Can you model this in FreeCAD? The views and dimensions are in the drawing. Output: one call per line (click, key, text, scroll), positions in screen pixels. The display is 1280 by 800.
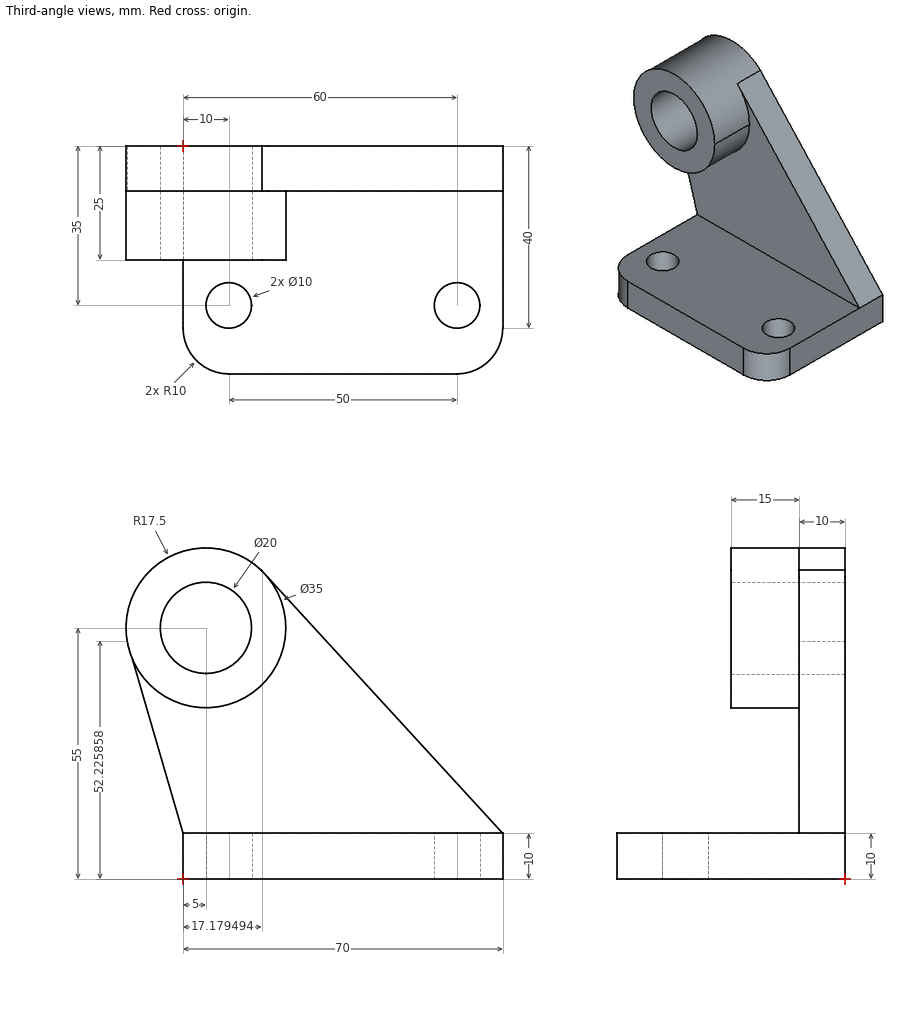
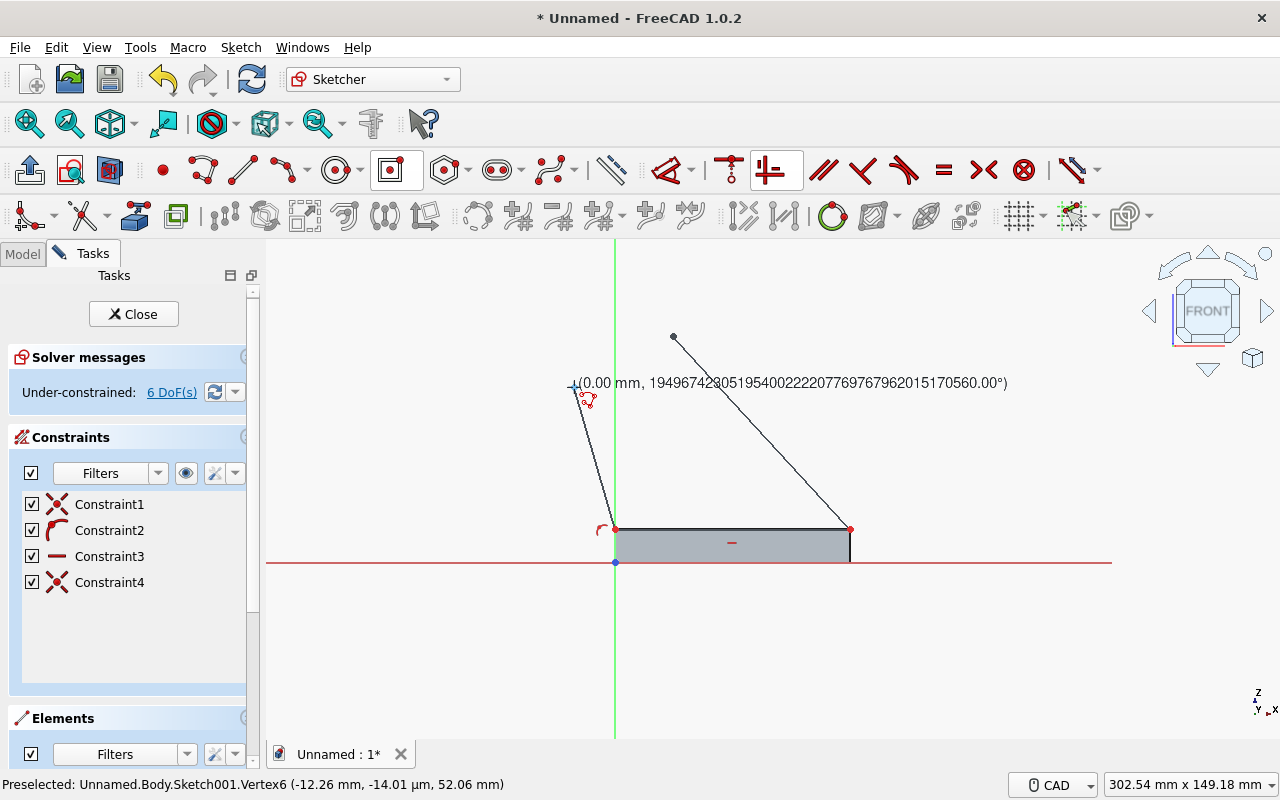
click(284, 170)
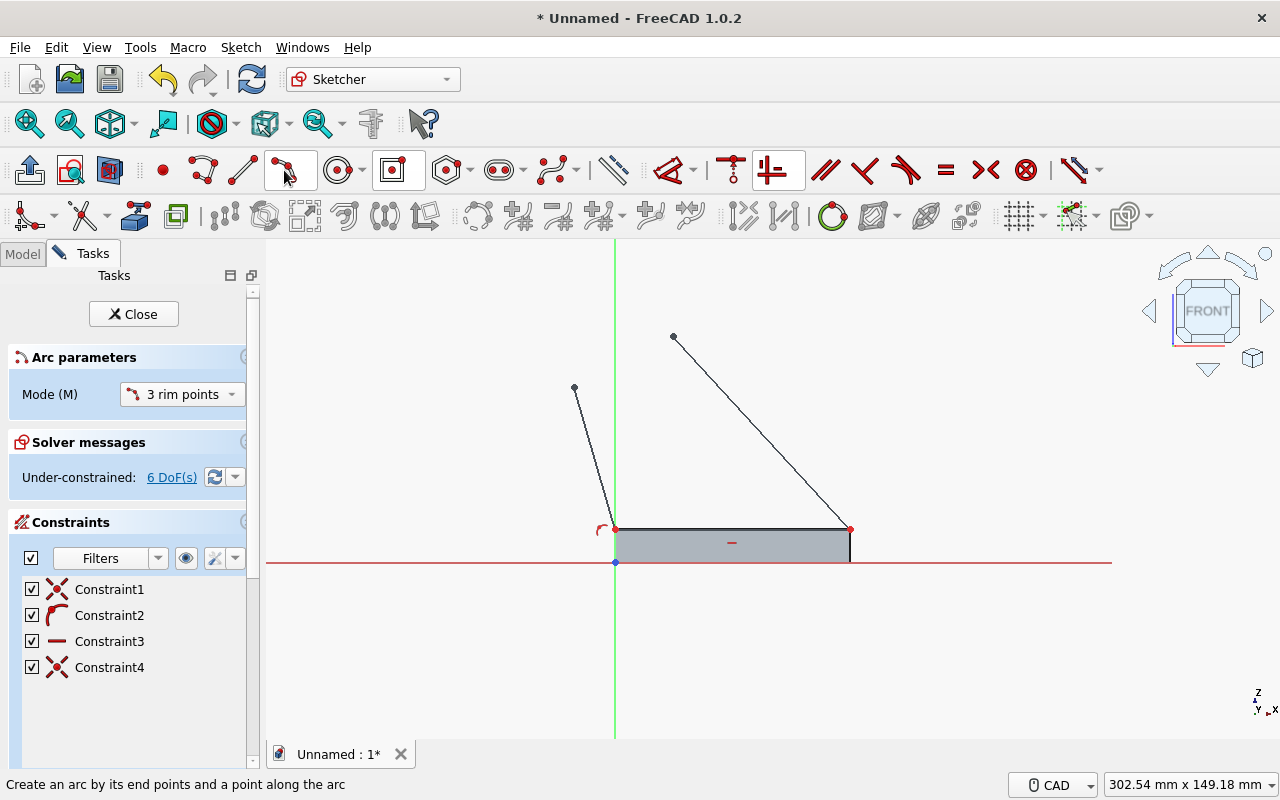
click(574, 388)
click(673, 337)
click(593, 334)
key(Escape)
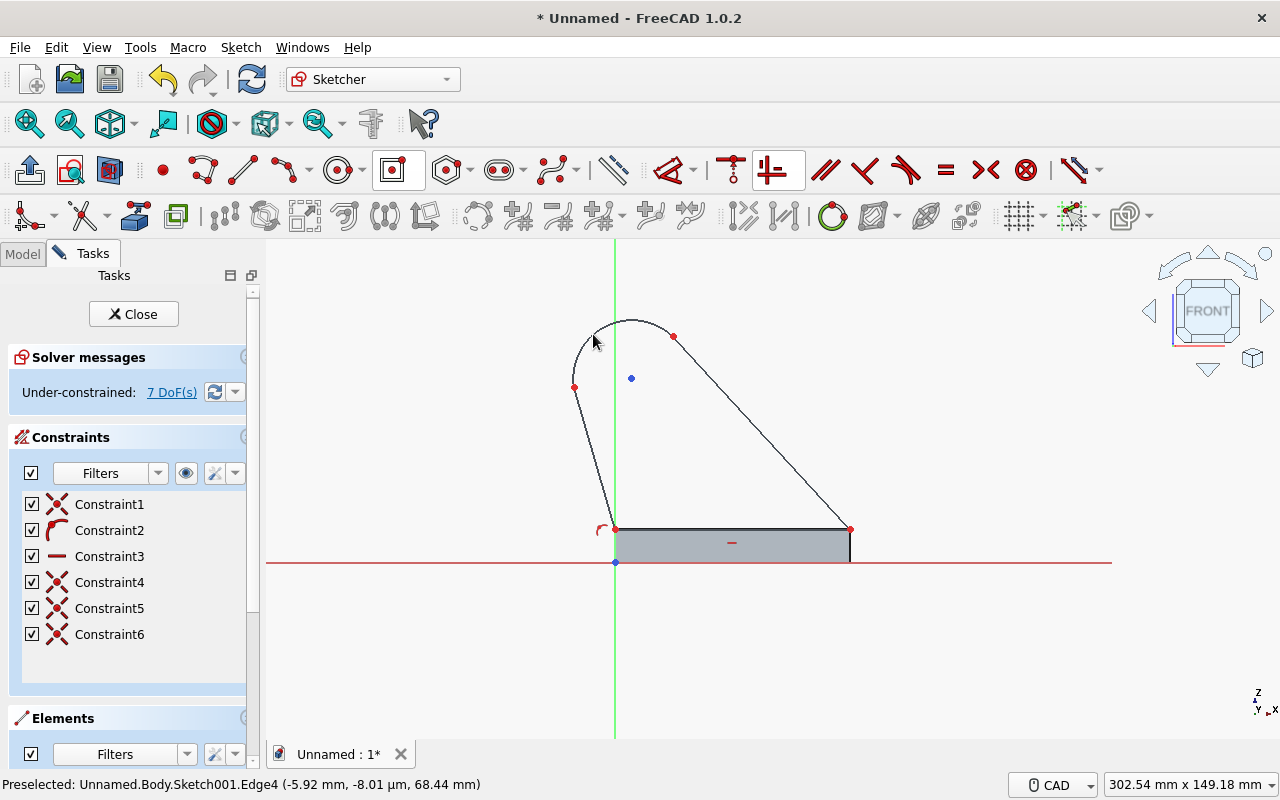
click(668, 170)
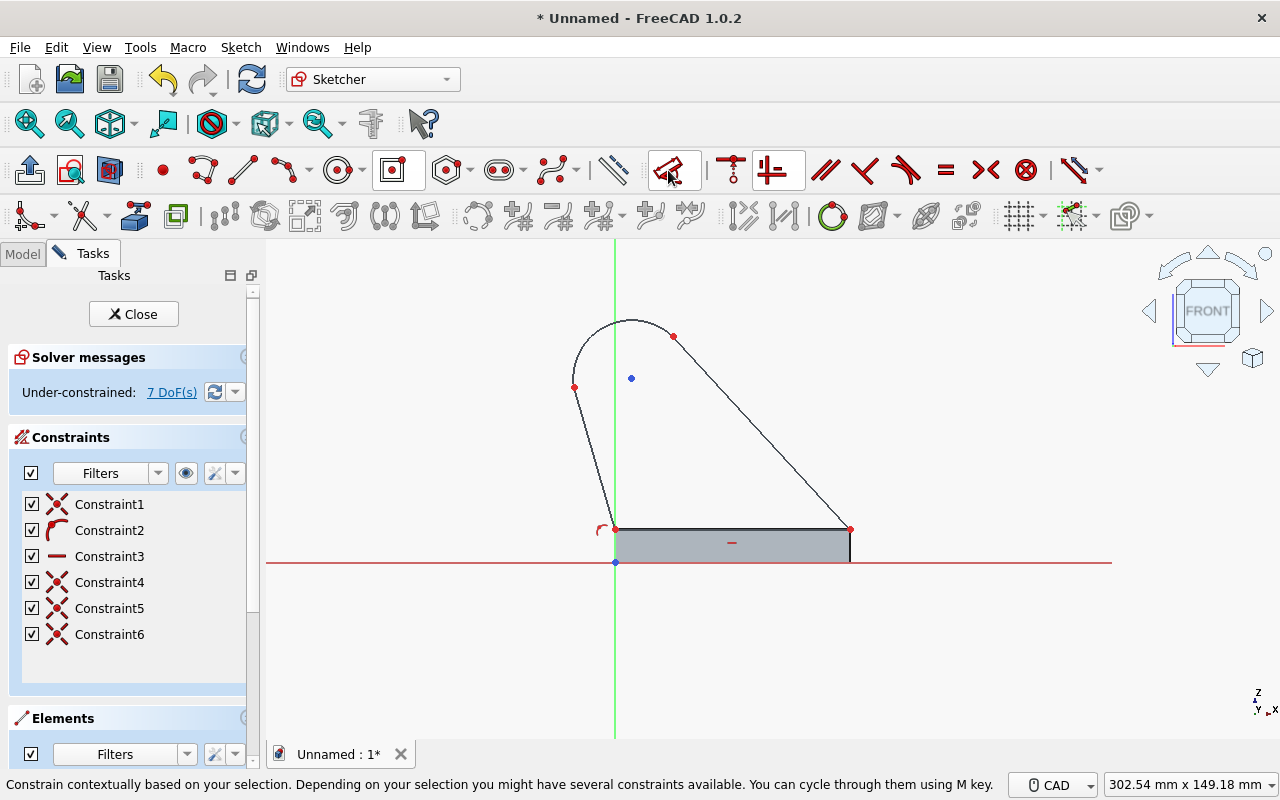
click(633, 320)
click(634, 288)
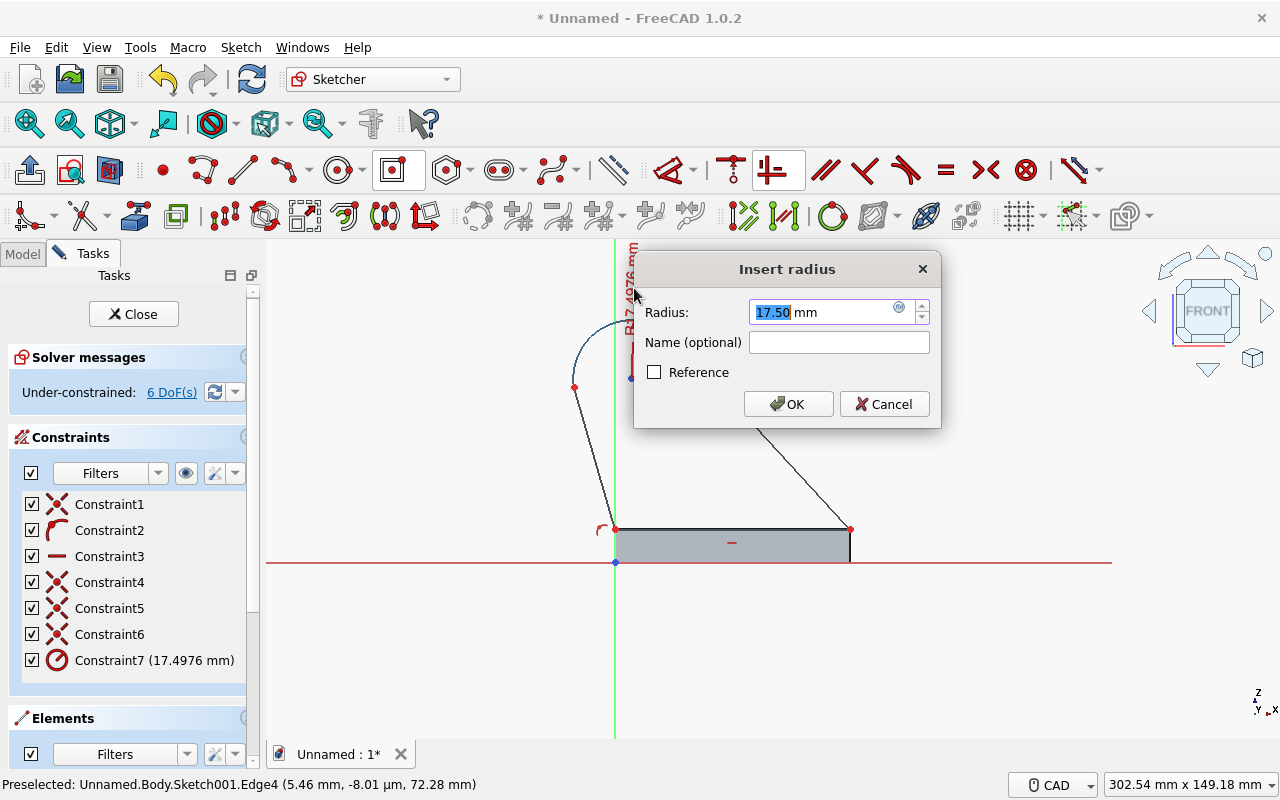
text(17.5)
key(Return)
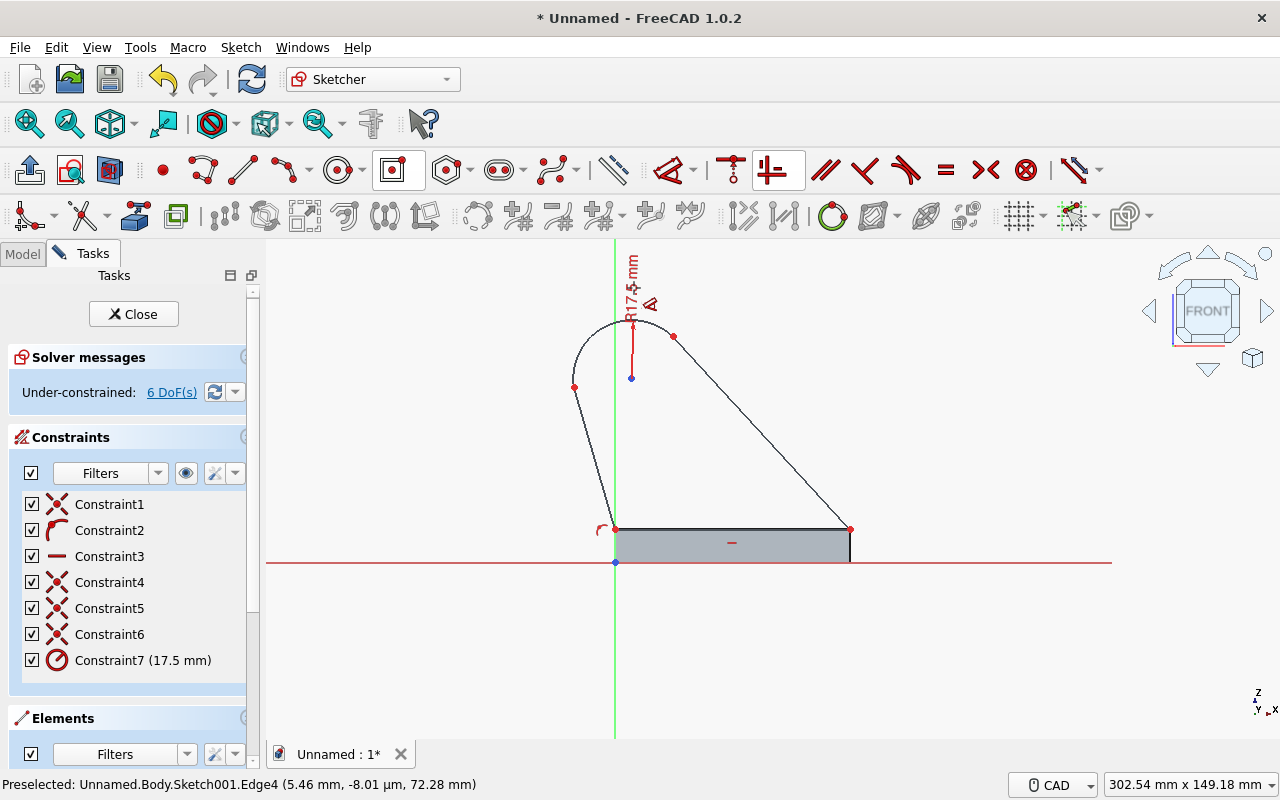
click(780, 530)
click(733, 496)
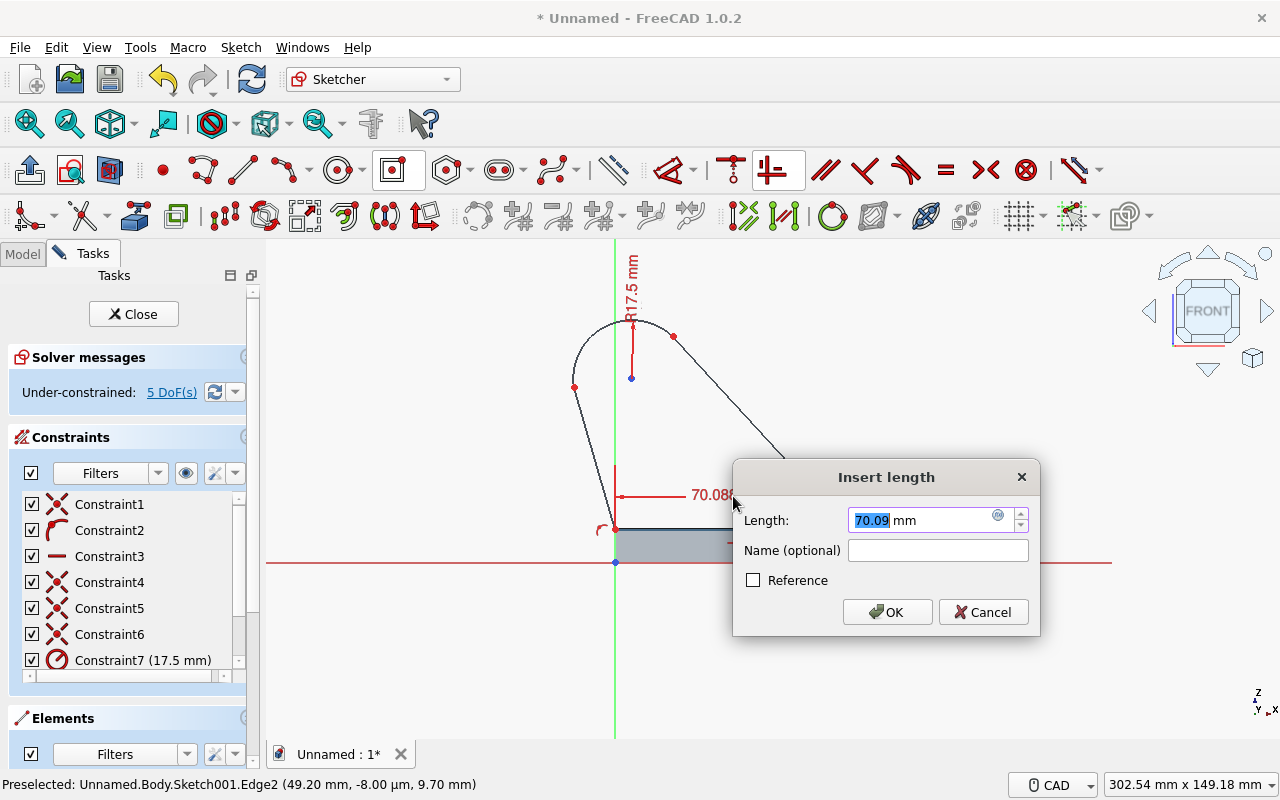
text(70)
key(Return)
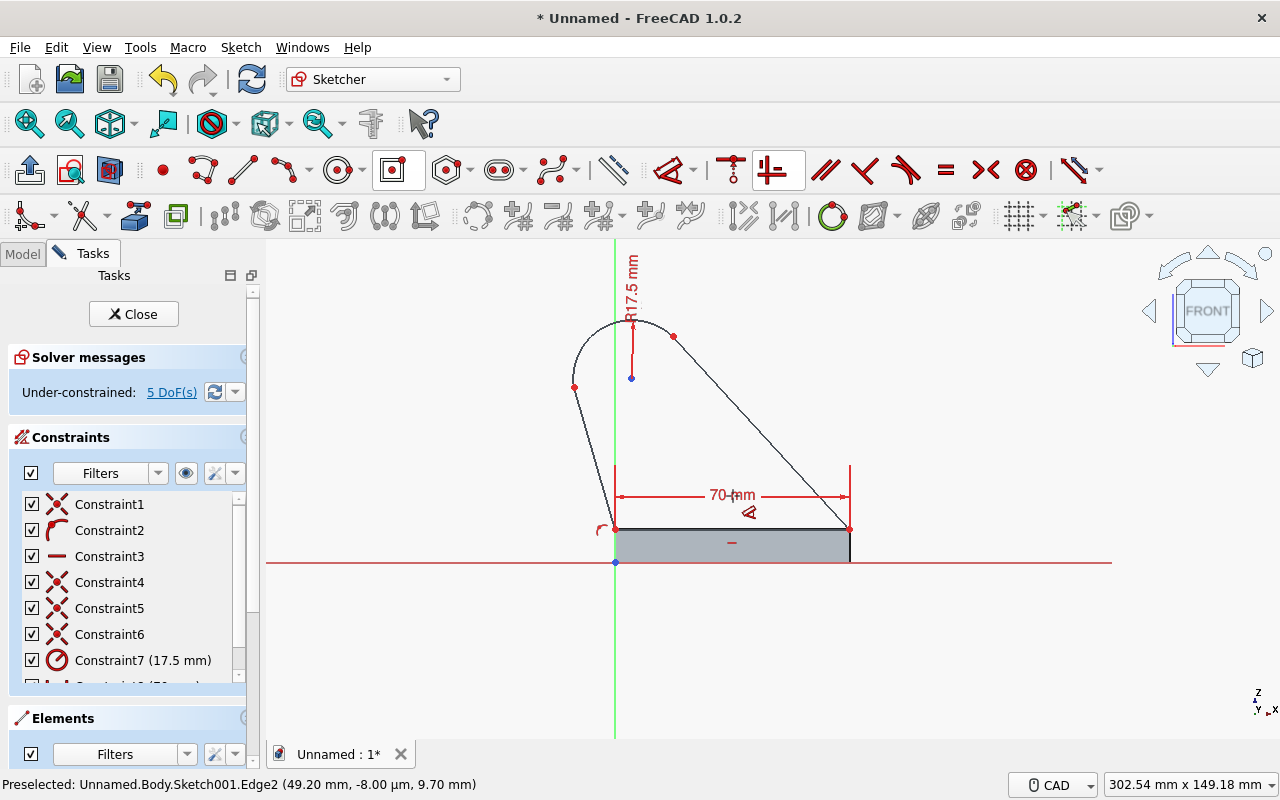
scroll(632, 379, up, 5)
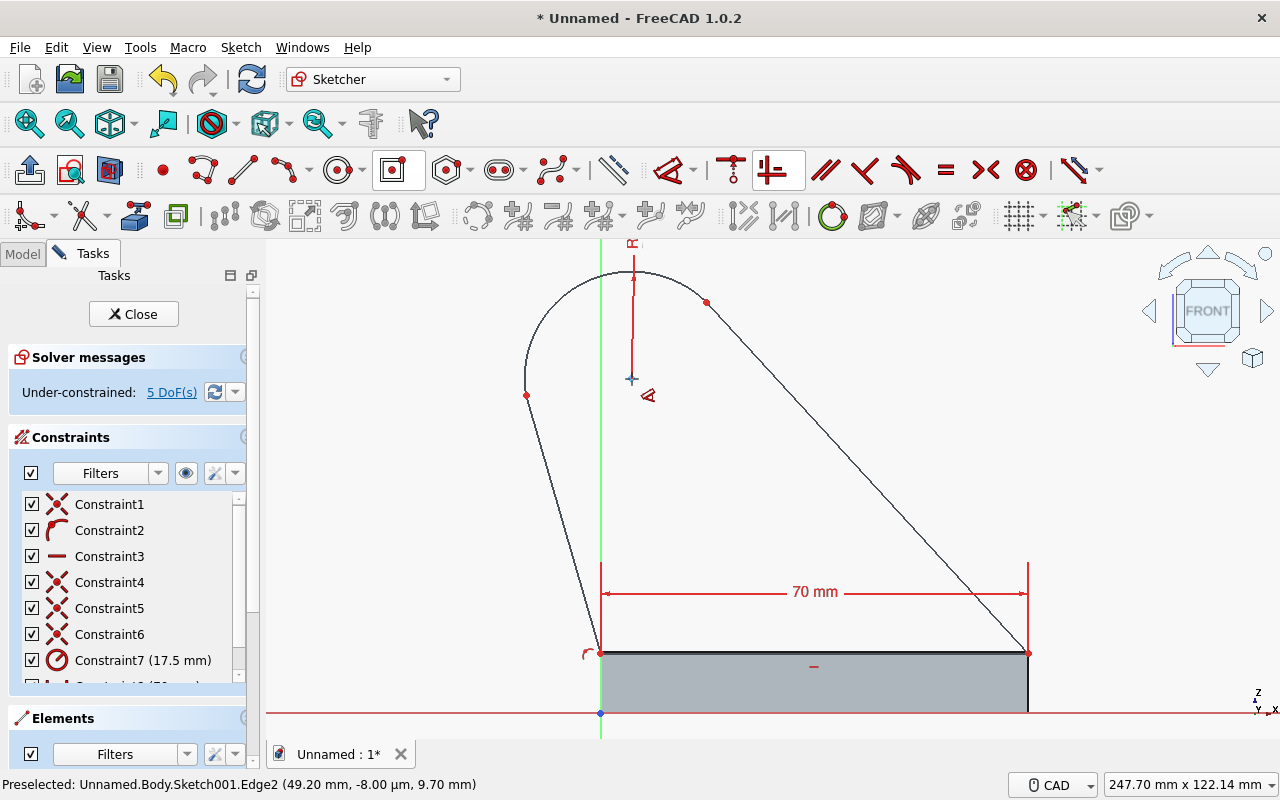
click(631, 378)
click(608, 344)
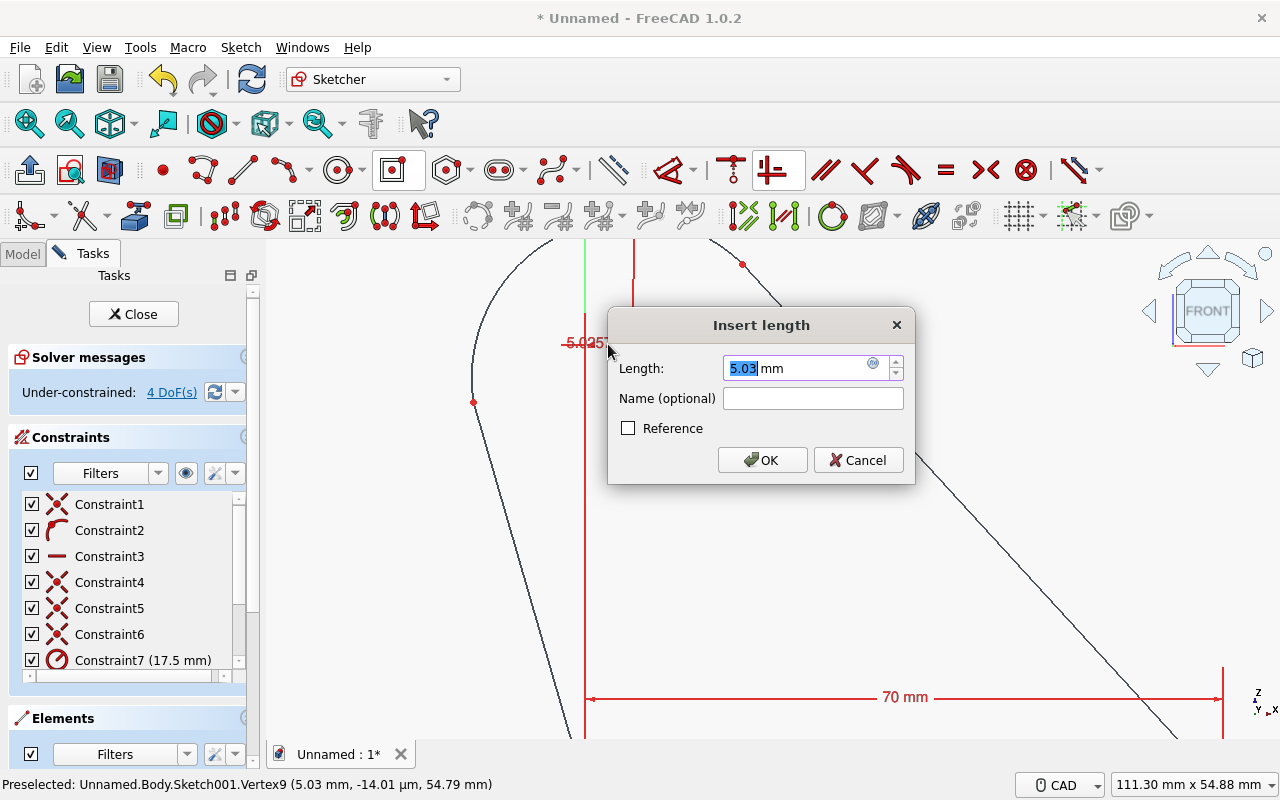
text(5)
key(Return)